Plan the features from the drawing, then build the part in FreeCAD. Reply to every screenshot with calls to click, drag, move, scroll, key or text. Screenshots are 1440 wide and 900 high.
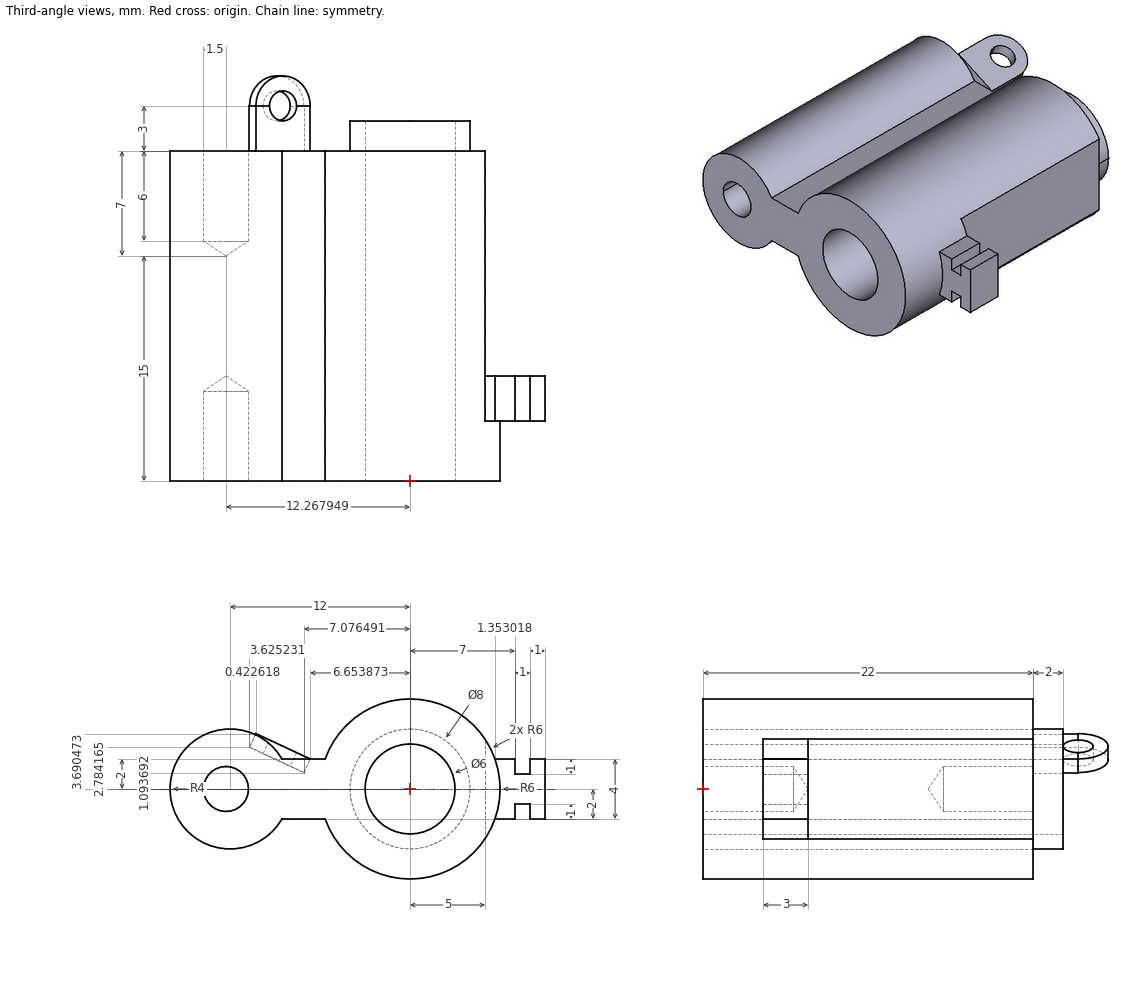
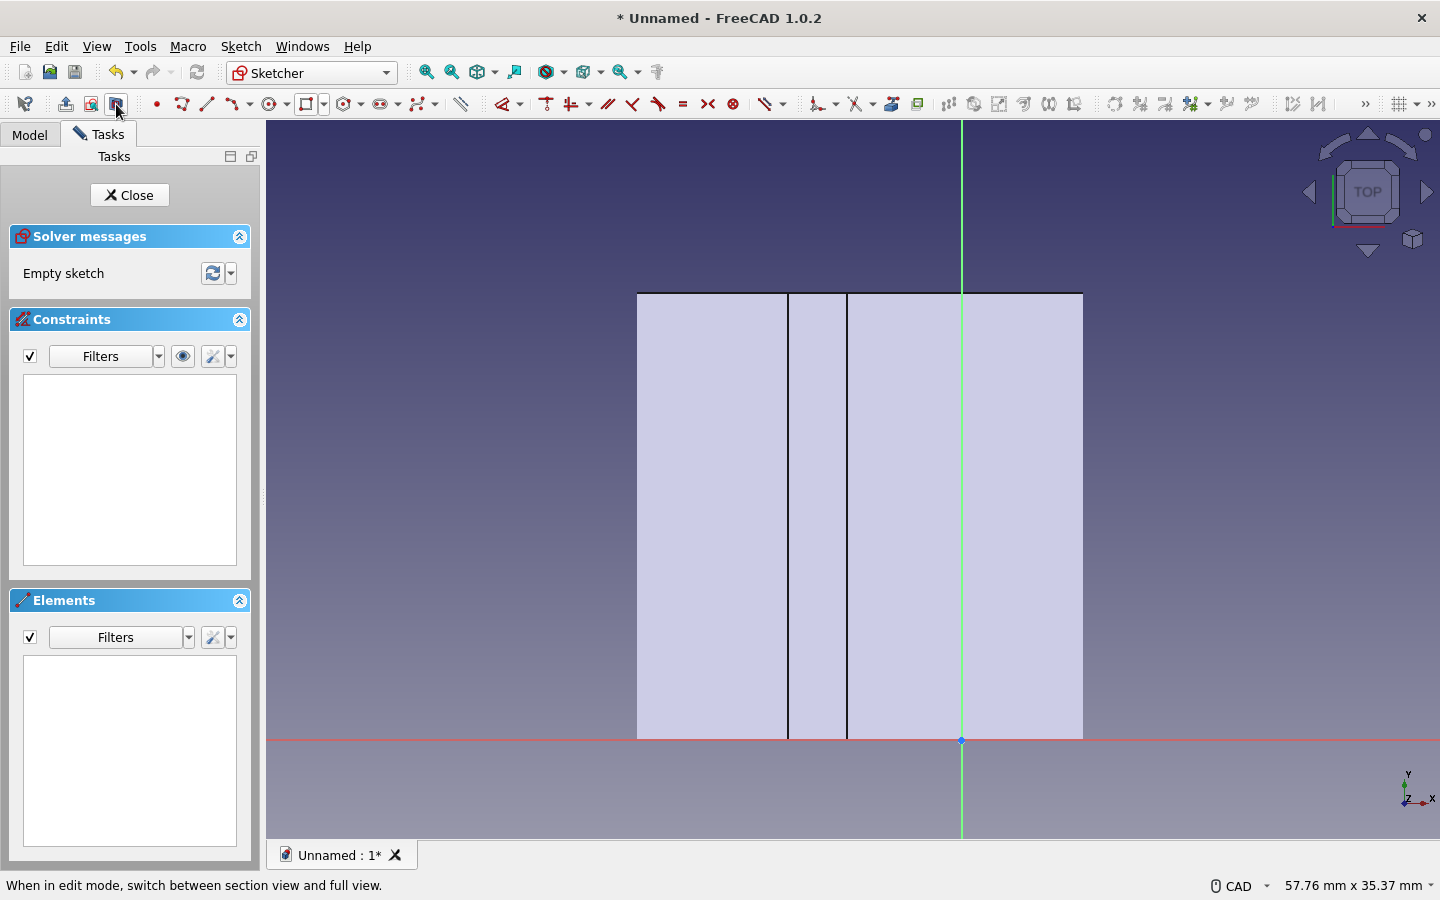
click(182, 104)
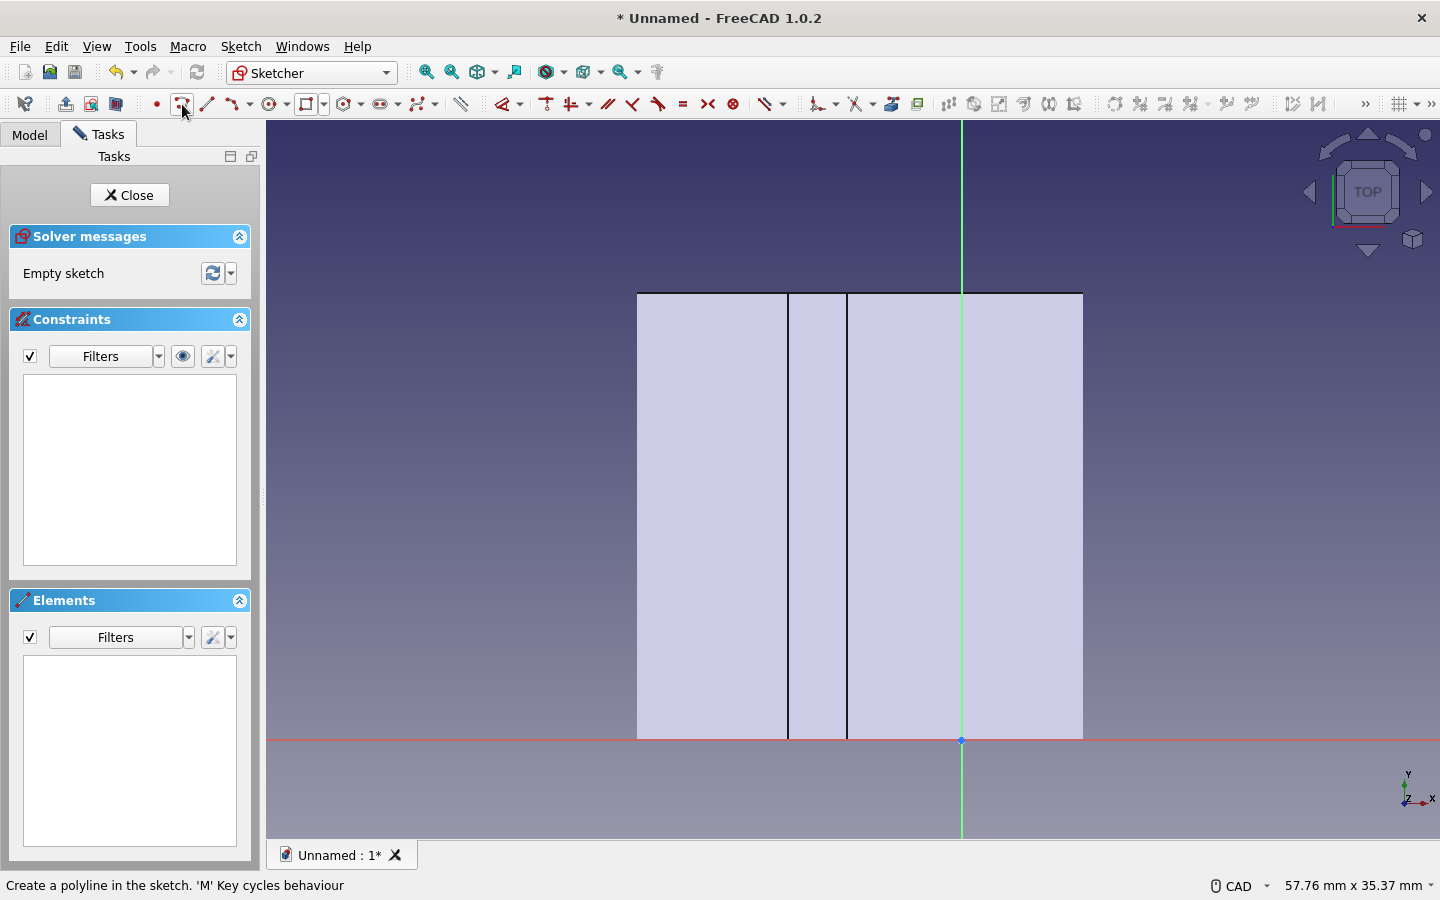
click(712, 436)
click(712, 293)
click(682, 293)
click(682, 415)
click(712, 437)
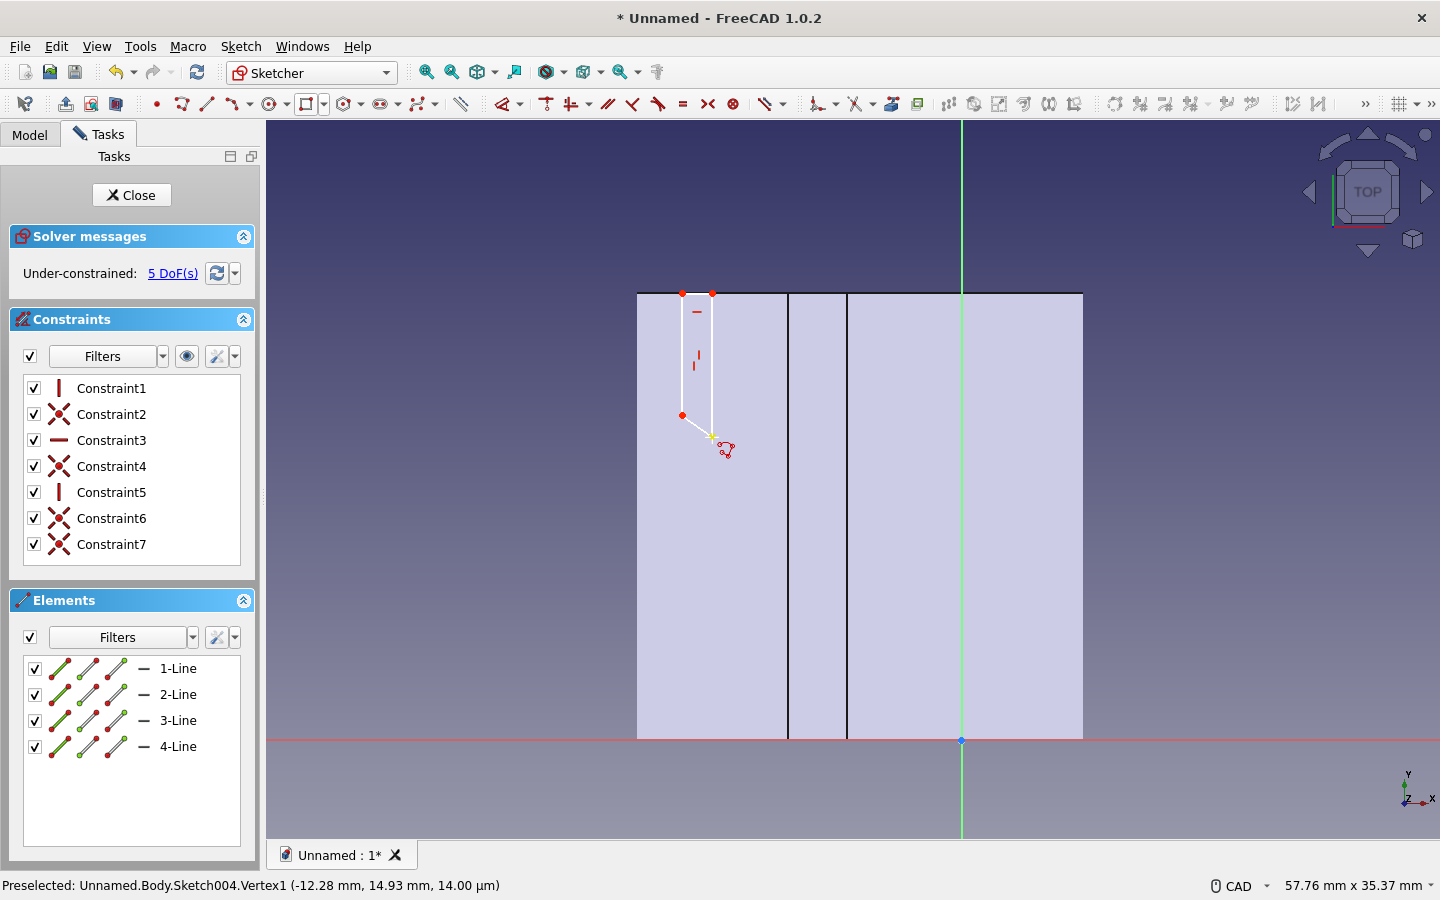
click(207, 104)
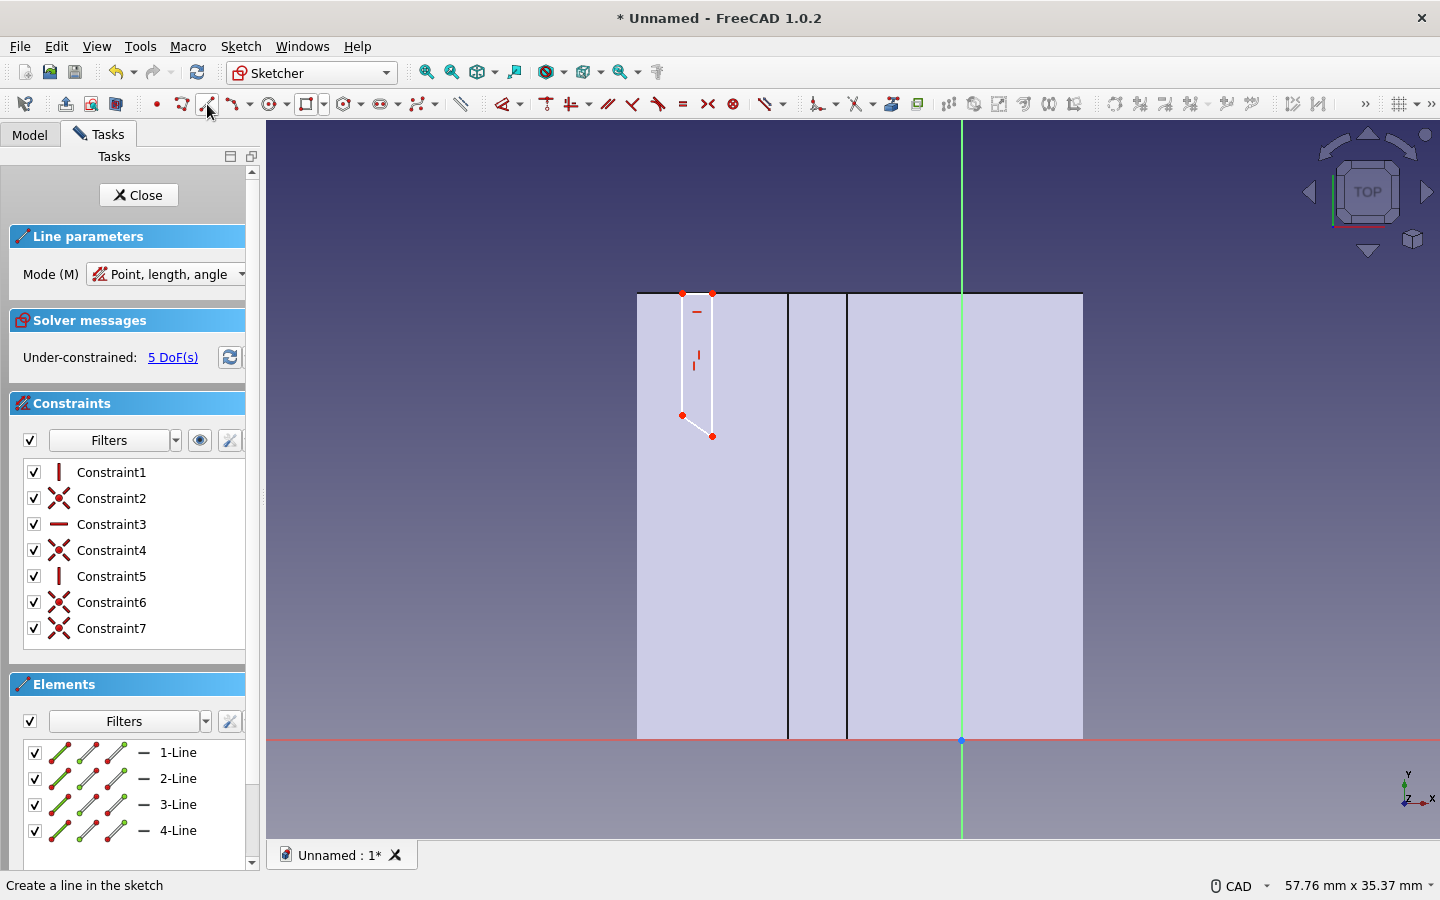
click(712, 450)
click(712, 492)
key(Escape)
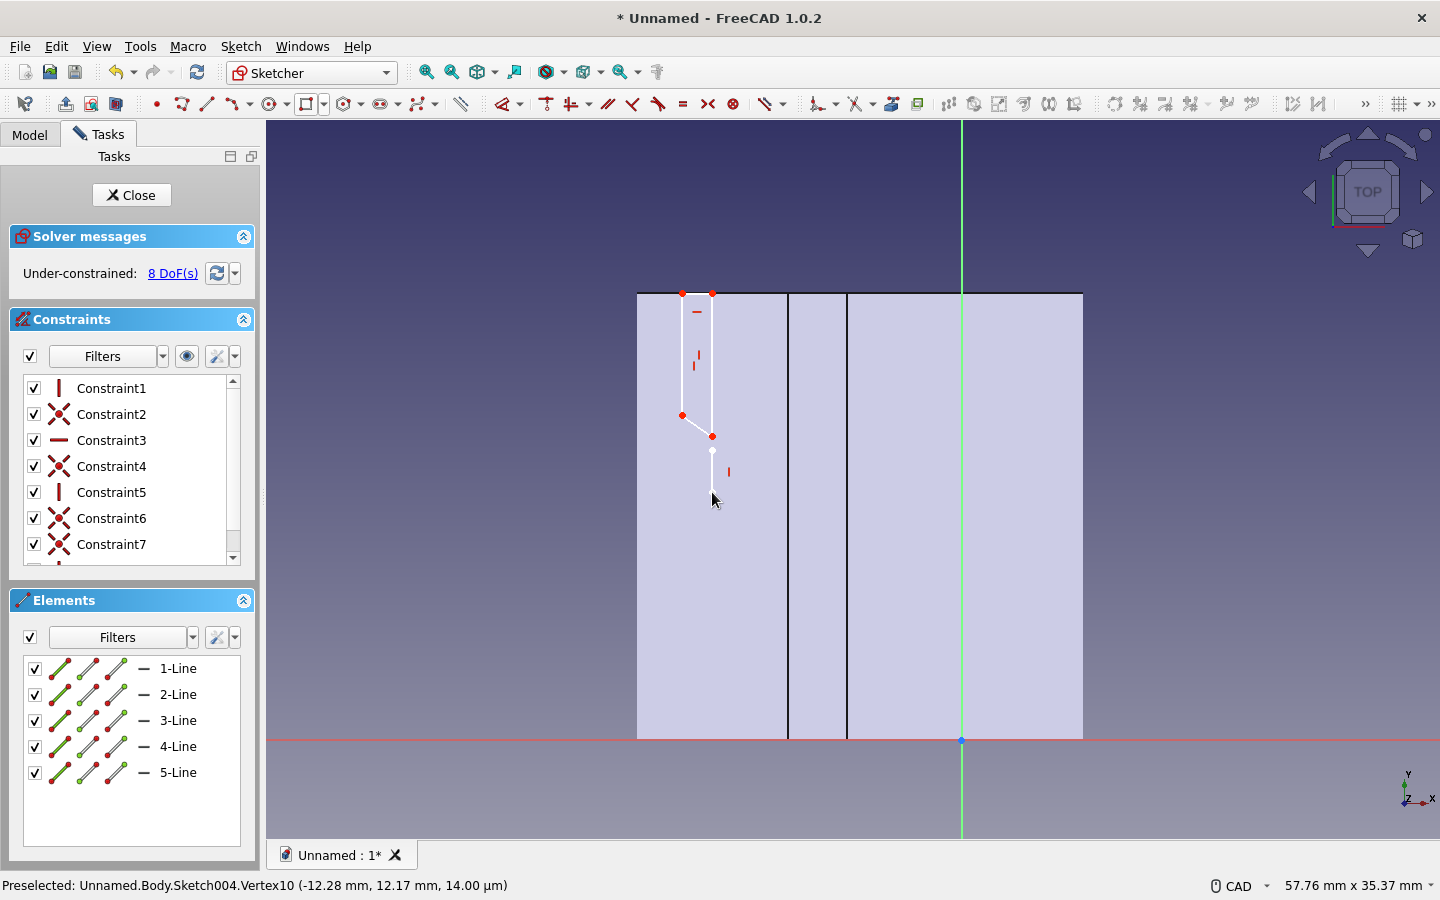
click(712, 464)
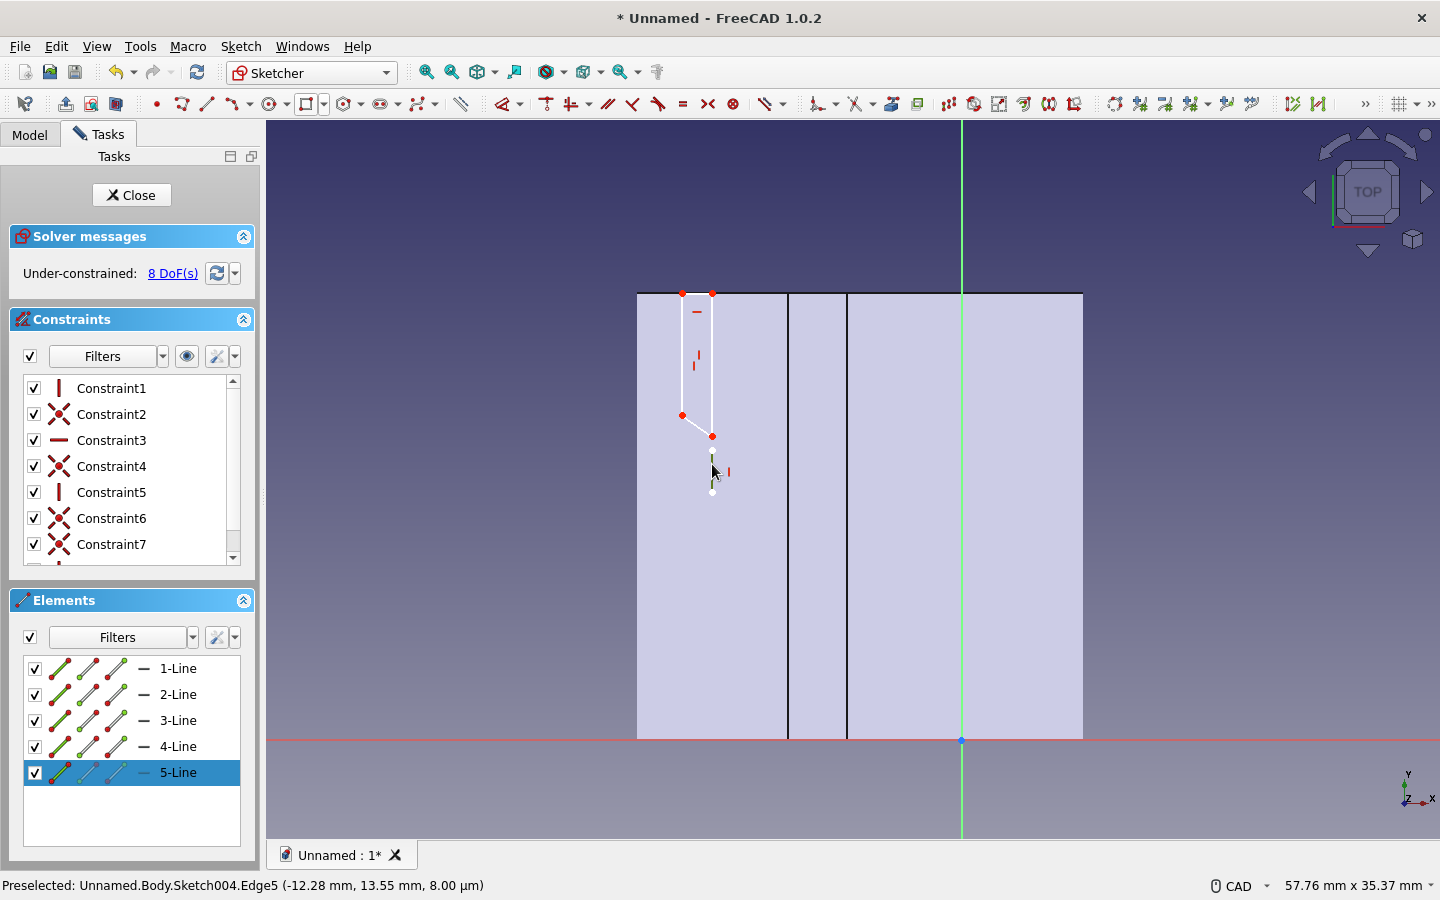
click(461, 104)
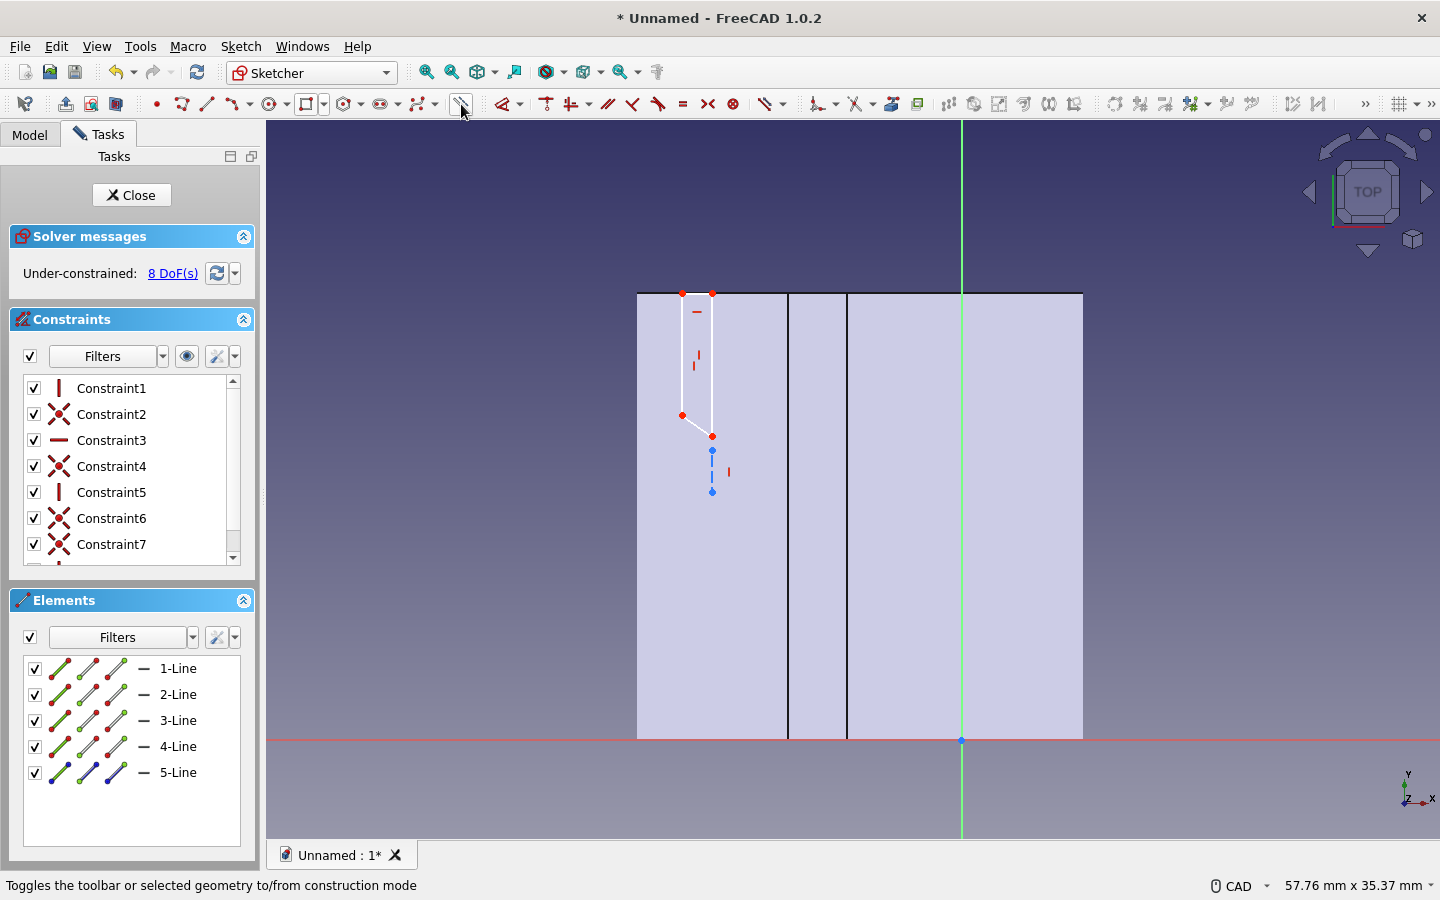
click(502, 104)